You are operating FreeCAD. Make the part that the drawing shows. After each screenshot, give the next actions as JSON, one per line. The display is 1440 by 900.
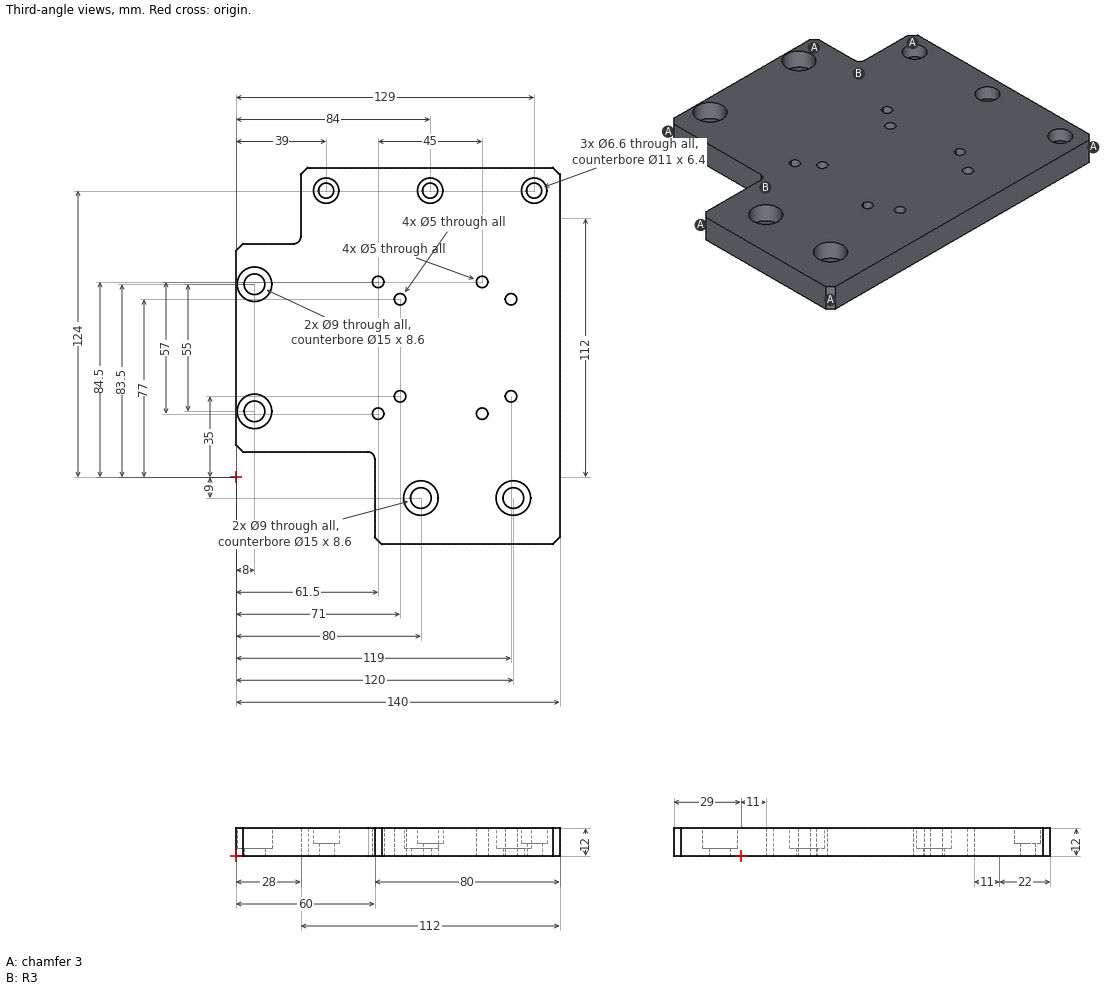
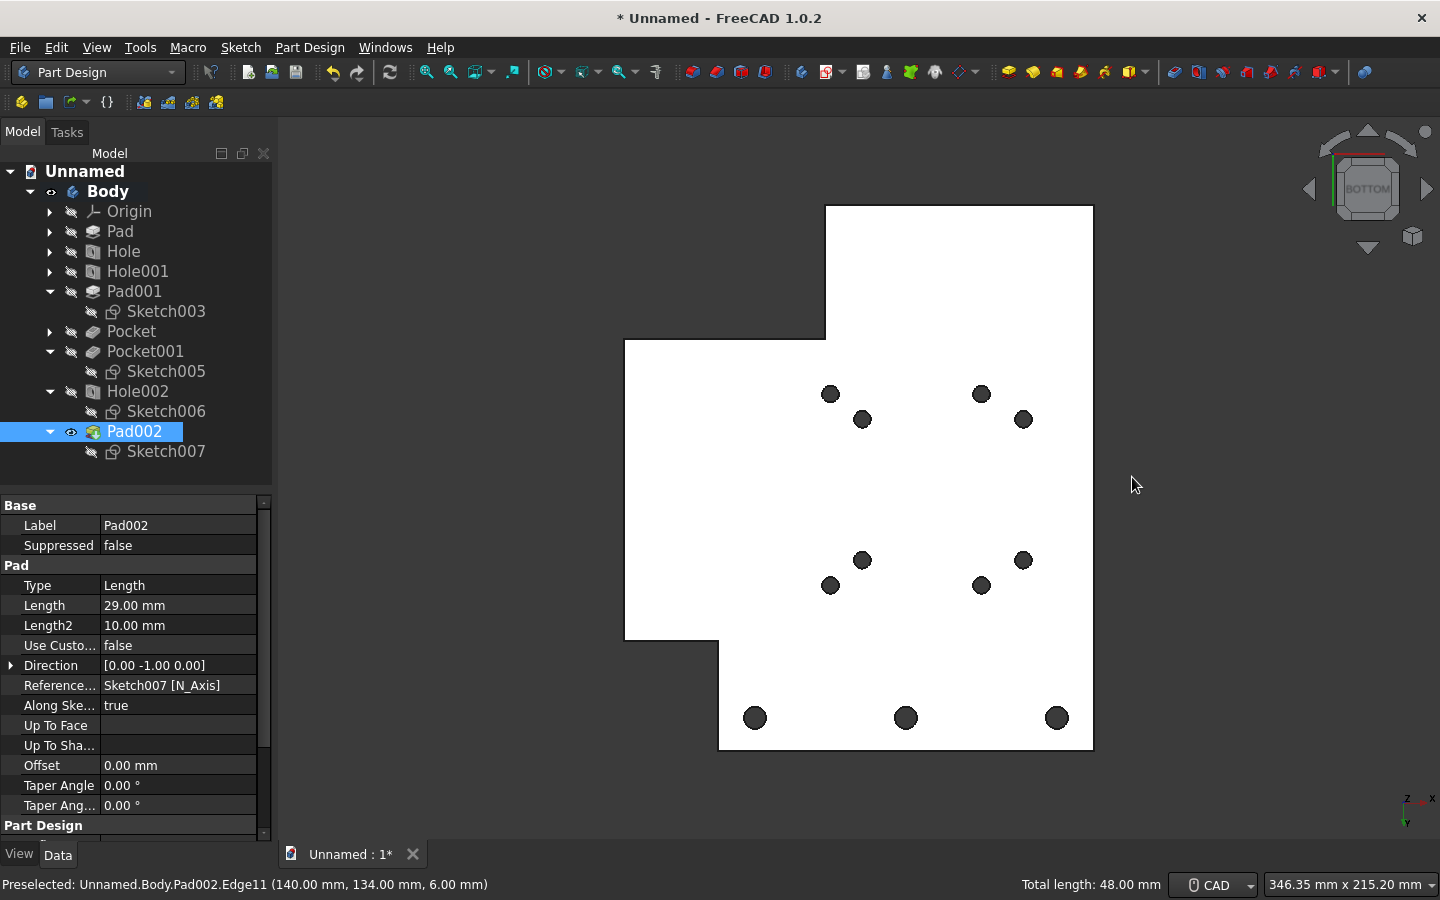
{"action": "key", "text": "4"}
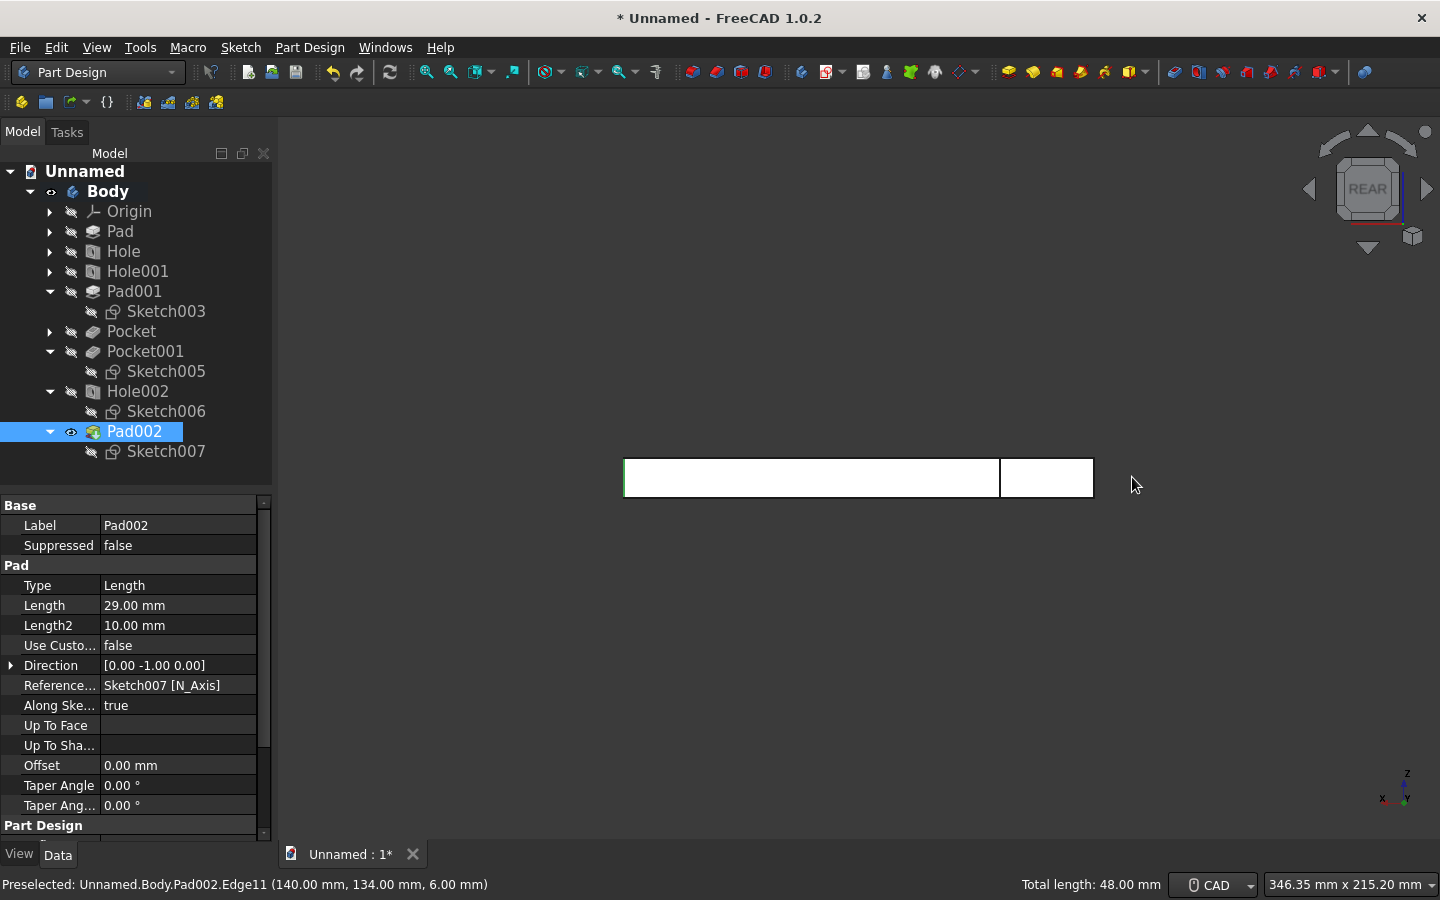
{"action": "key", "text": "v f"}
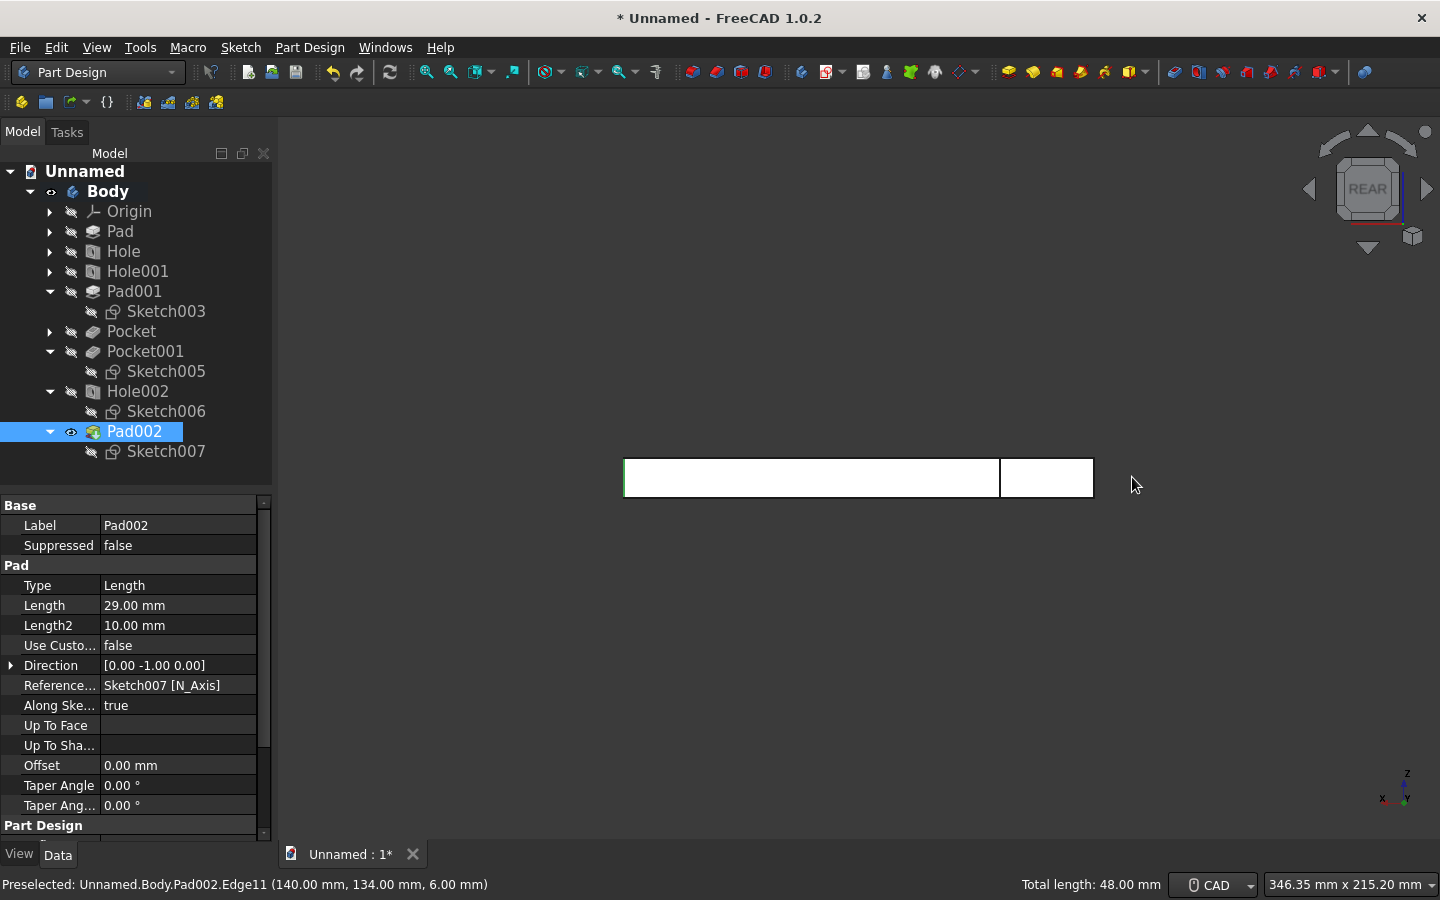
{"action": "left_click", "coordinate": [1094, 477], "text": "ctrl"}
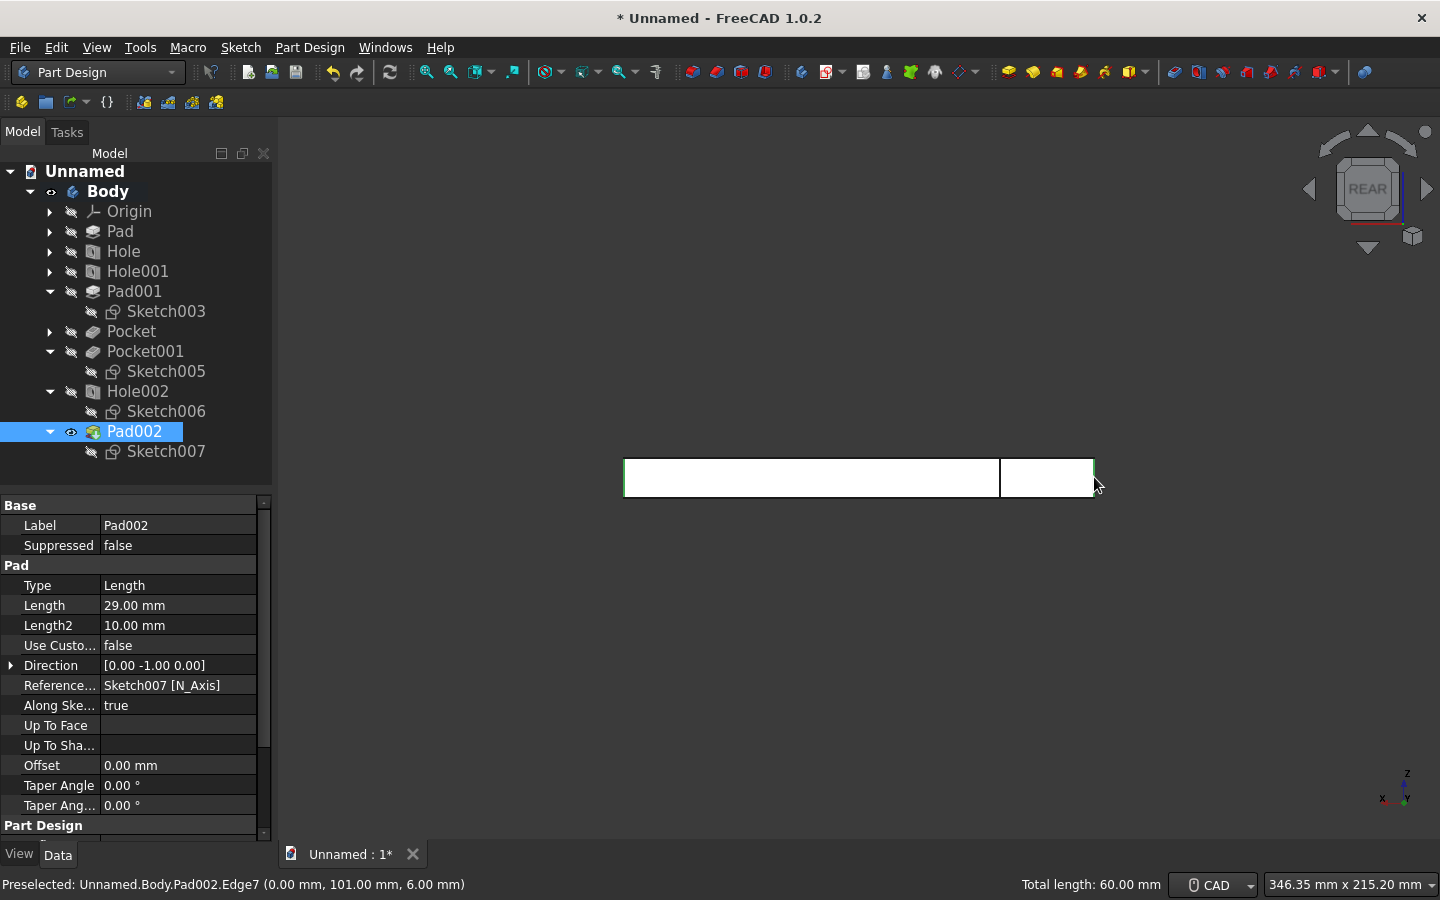
{"action": "left_click", "coordinate": [1000, 477], "text": "ctrl"}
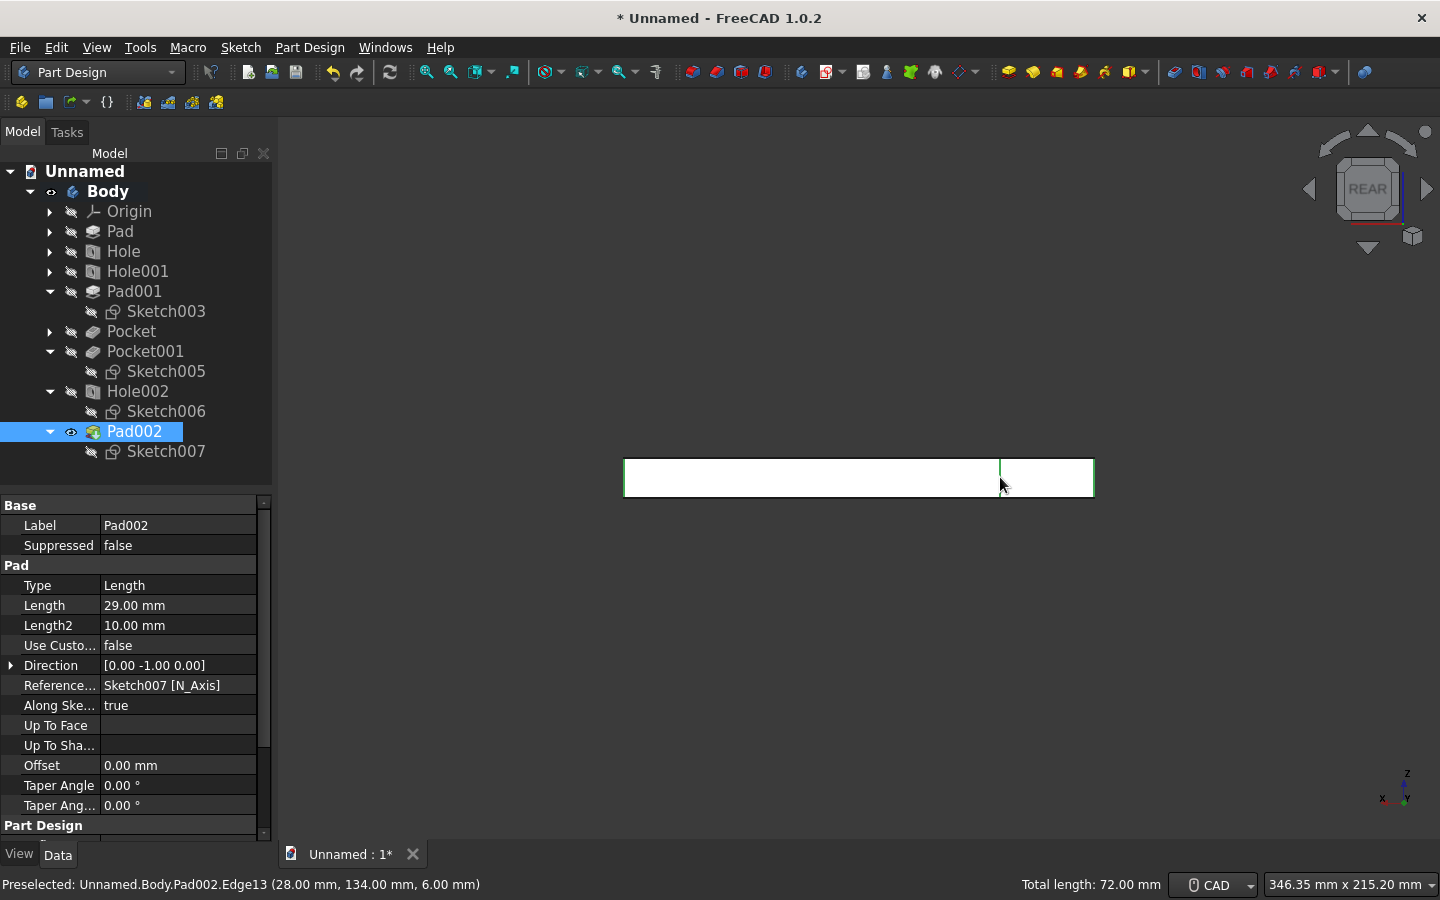
{"action": "left_click", "coordinate": [718, 72]}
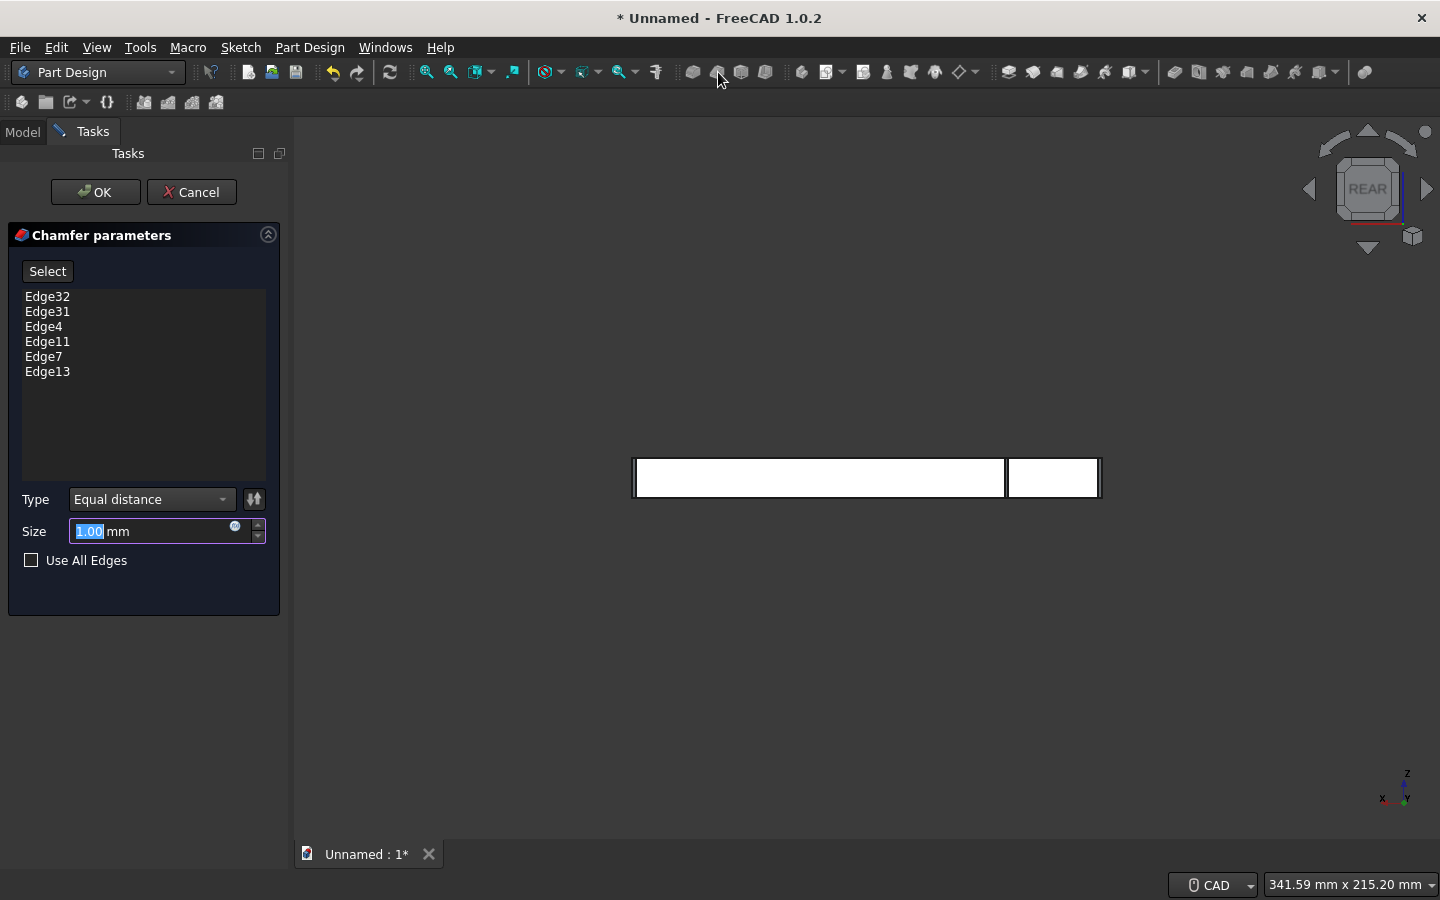
{"action": "type", "text": "3"}
{"action": "key", "text": "Tab"}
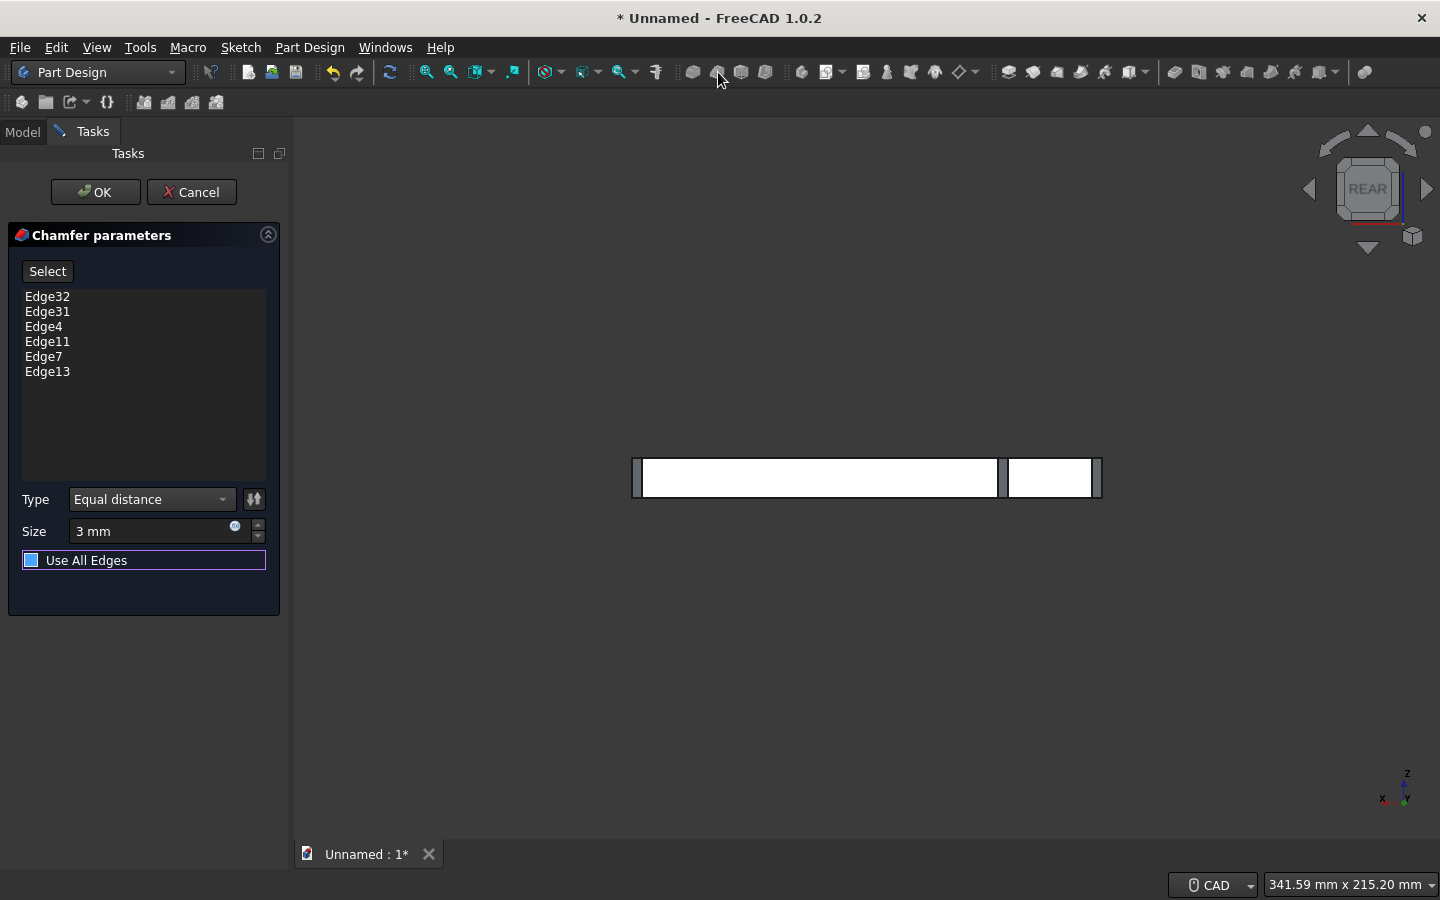
{"action": "left_click", "coordinate": [96, 192]}